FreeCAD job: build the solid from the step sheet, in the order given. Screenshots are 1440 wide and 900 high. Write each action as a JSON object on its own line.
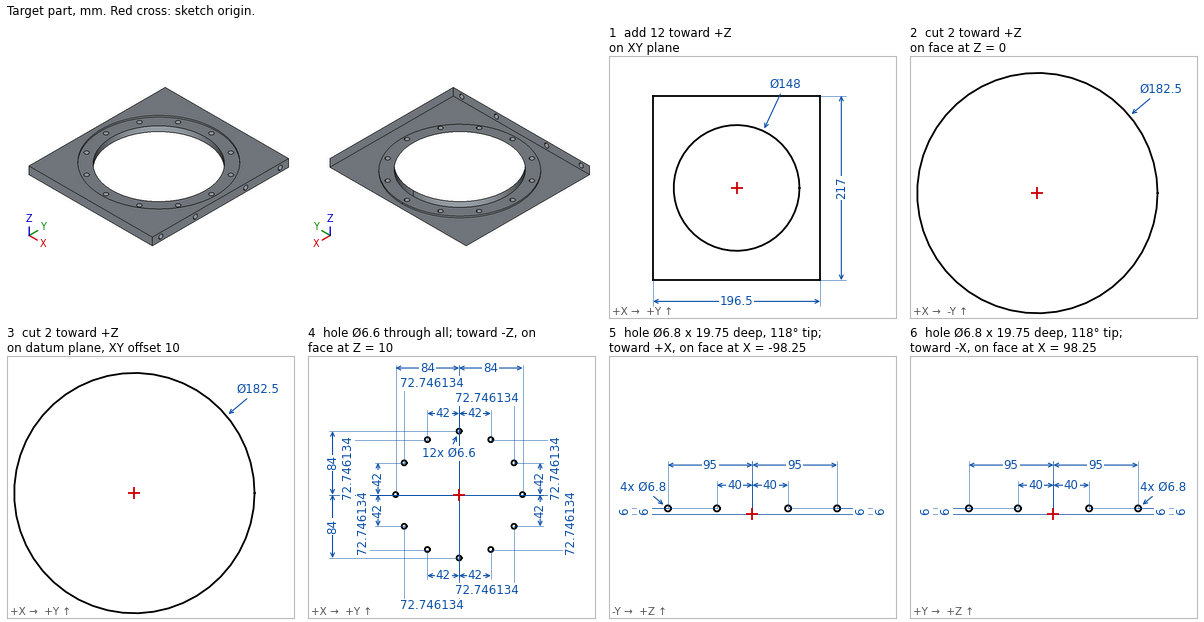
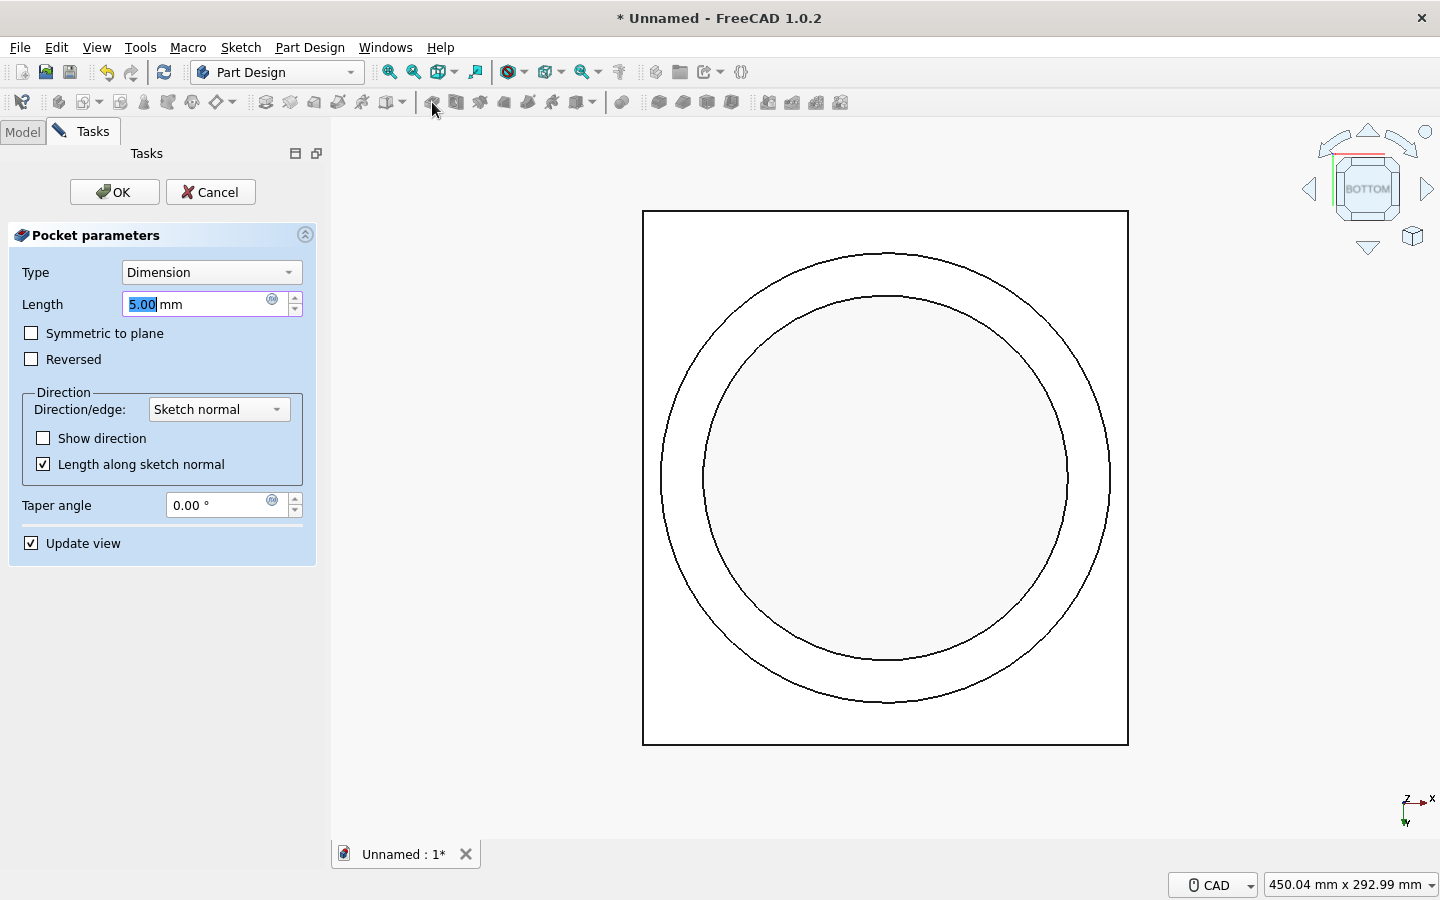
{"action": "type", "text": "2"}
{"action": "key", "text": "Tab"}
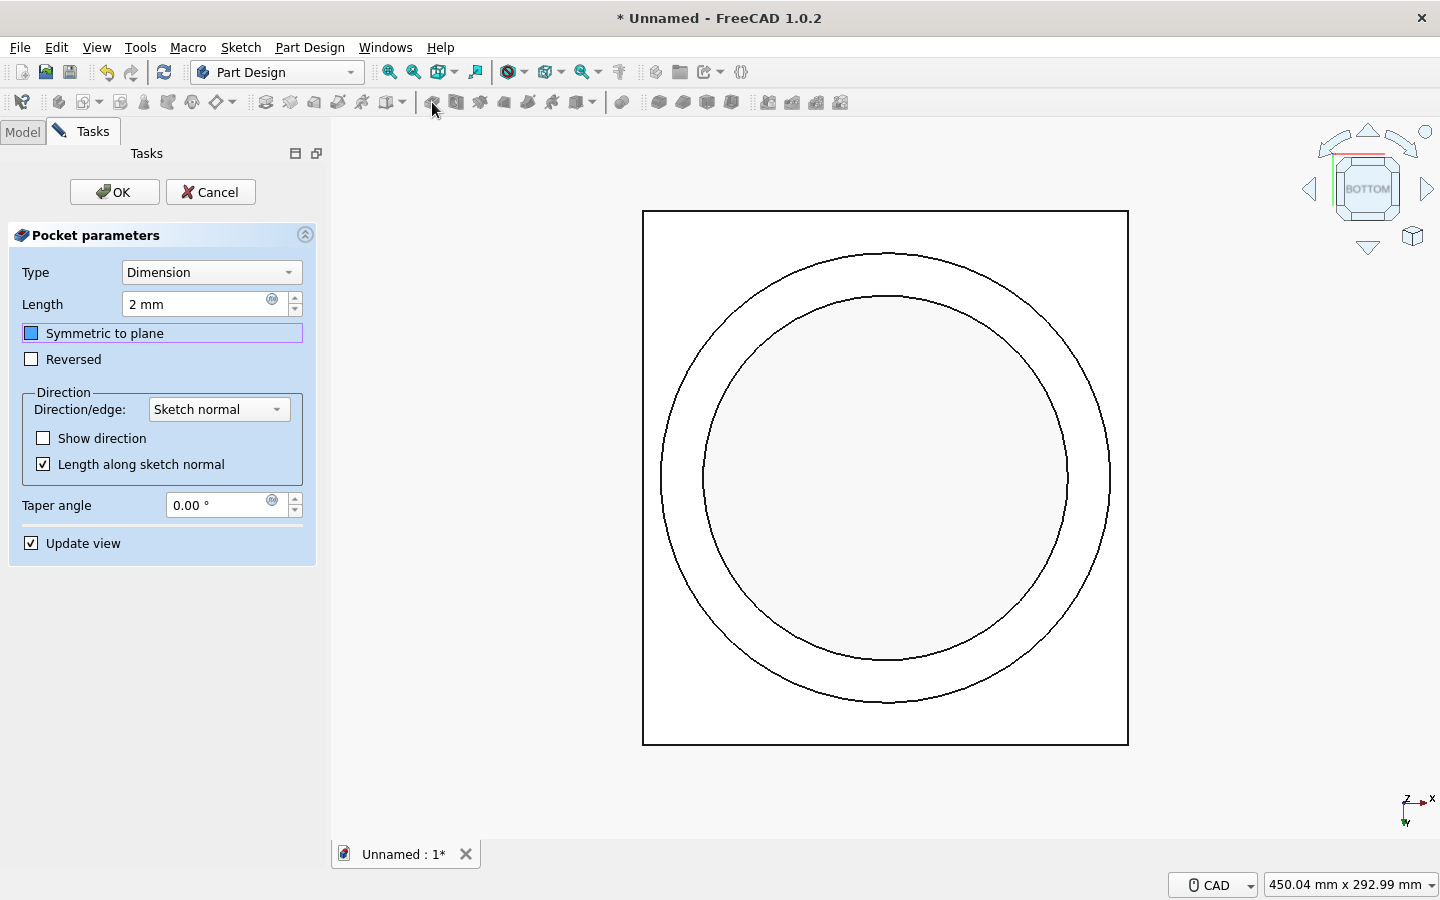
{"action": "left_click", "coordinate": [115, 192]}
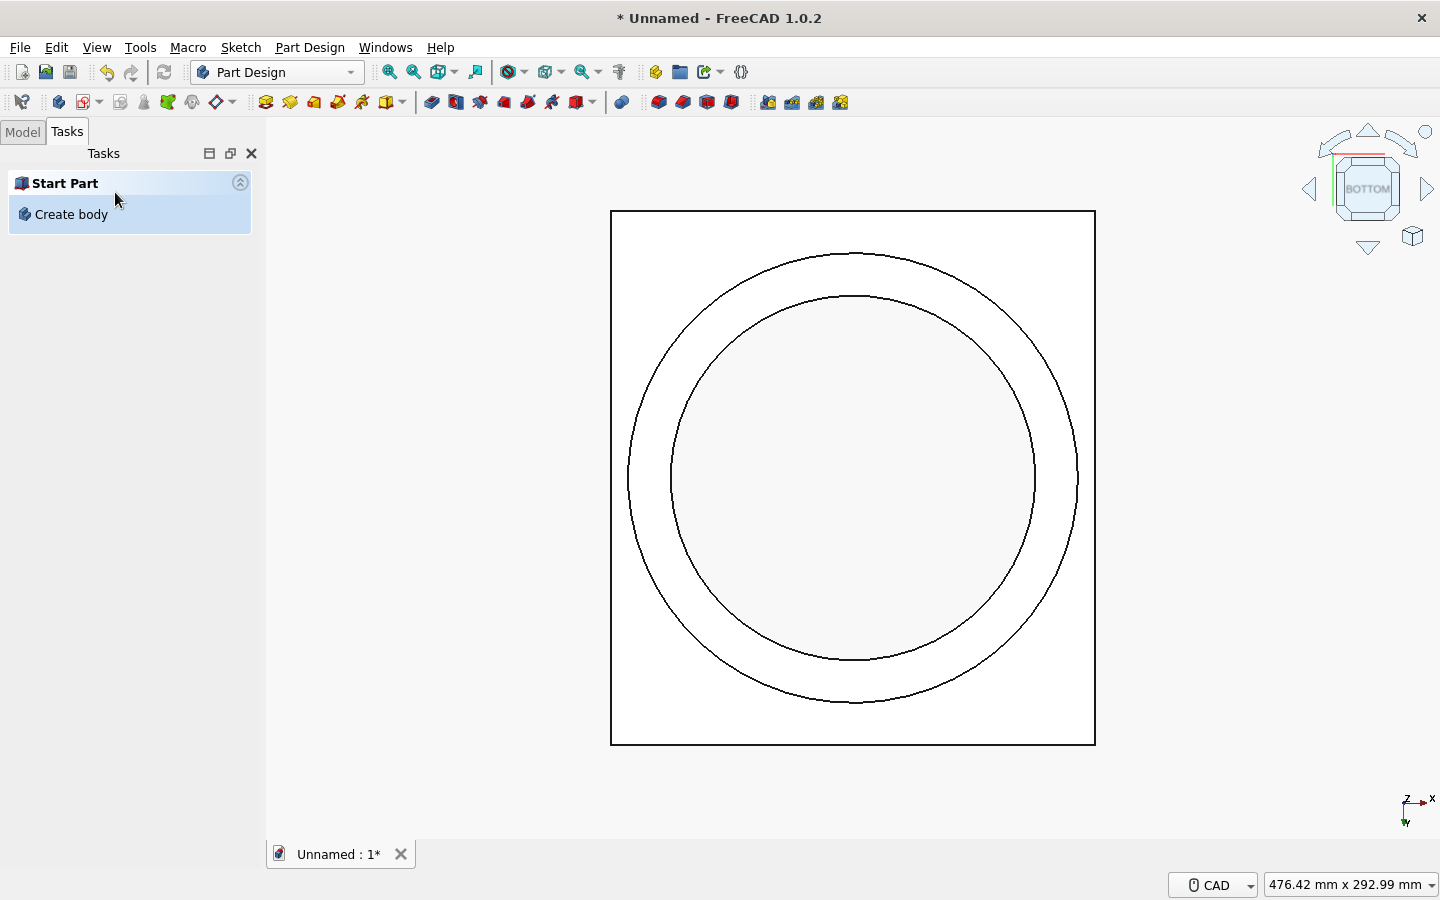
{"action": "left_click", "coordinate": [23, 131]}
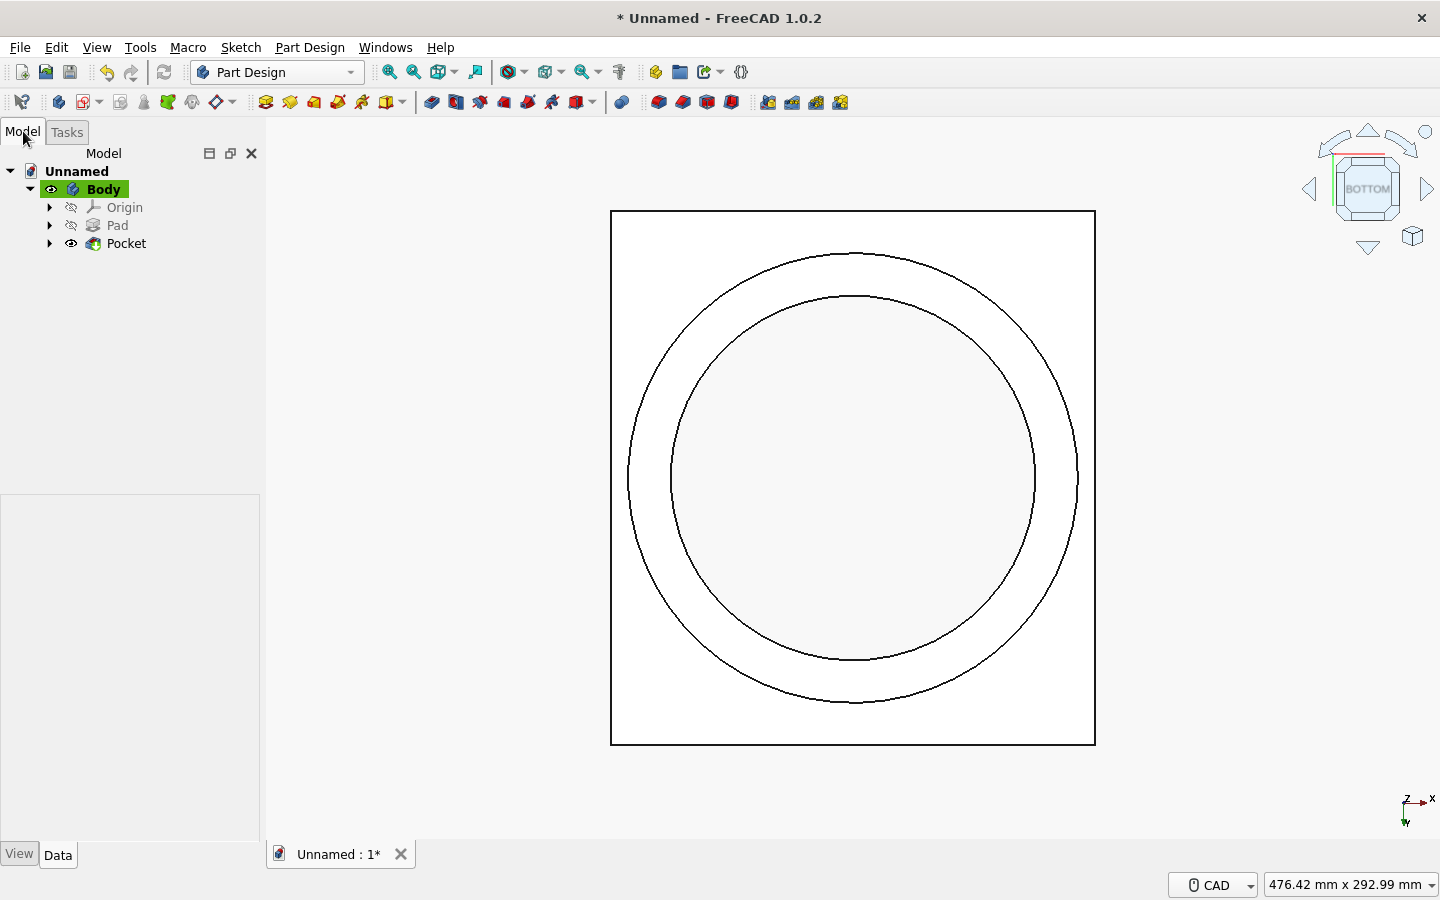
{"action": "left_click", "coordinate": [50, 207]}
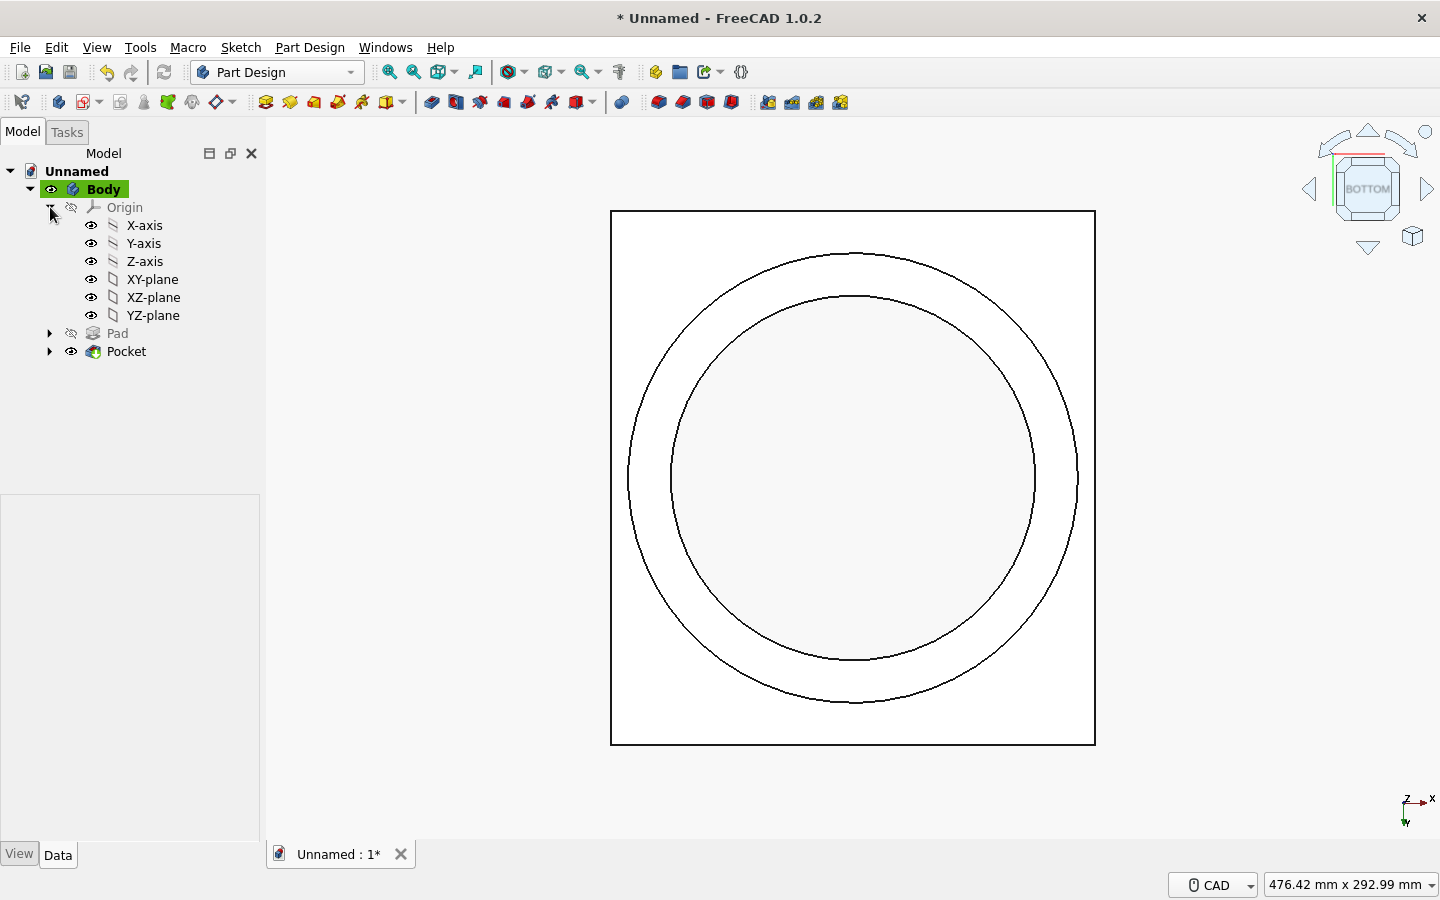
{"action": "left_click", "coordinate": [136, 279]}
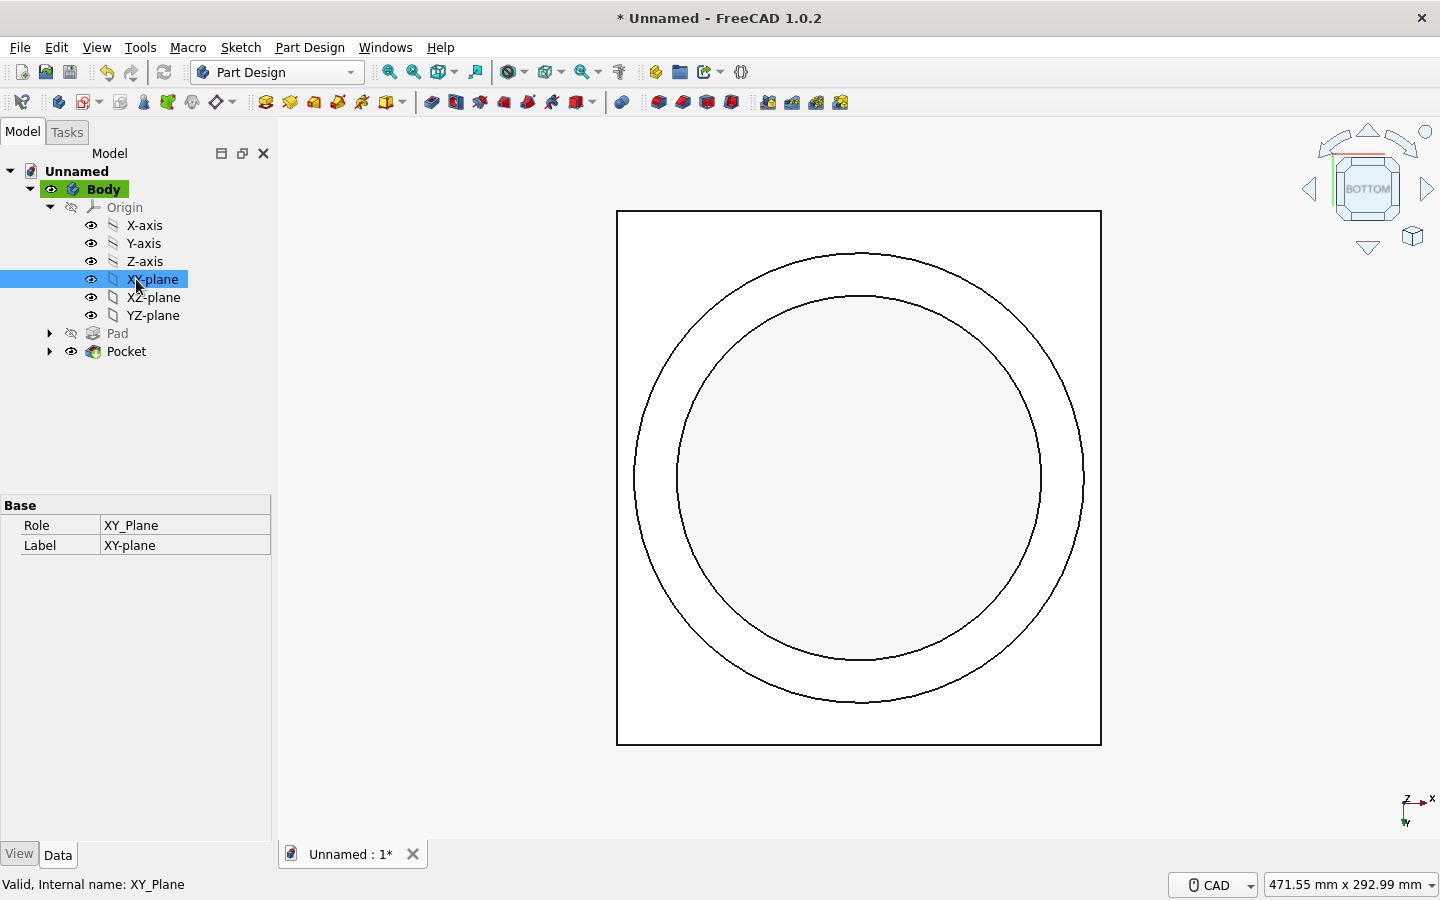
{"action": "left_click", "coordinate": [216, 102]}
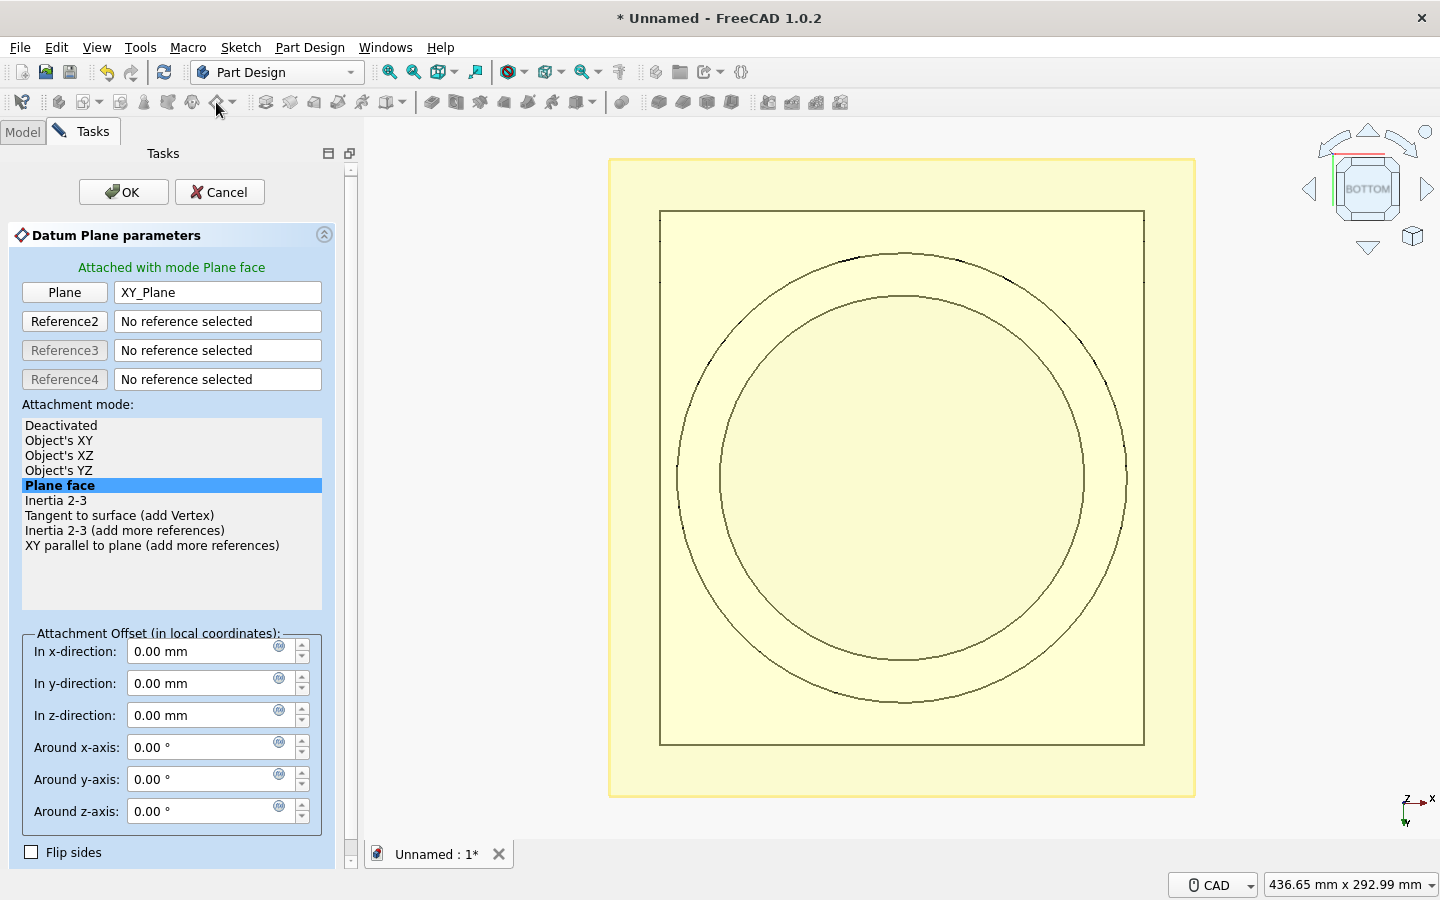
{"action": "triple_click", "coordinate": [210, 715]}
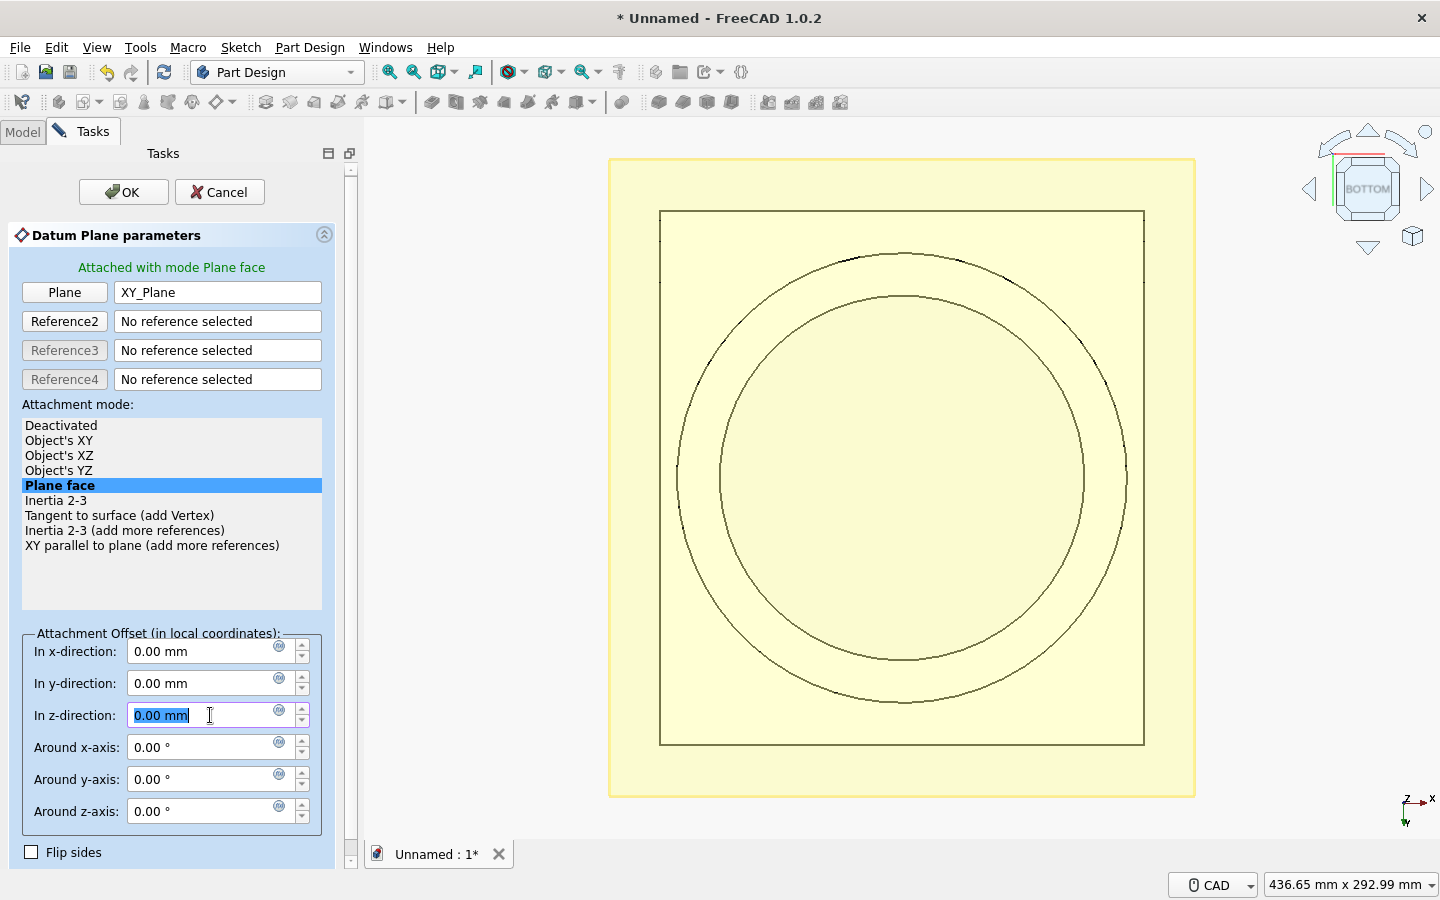
{"action": "type", "text": "10"}
{"action": "key", "text": "Tab"}